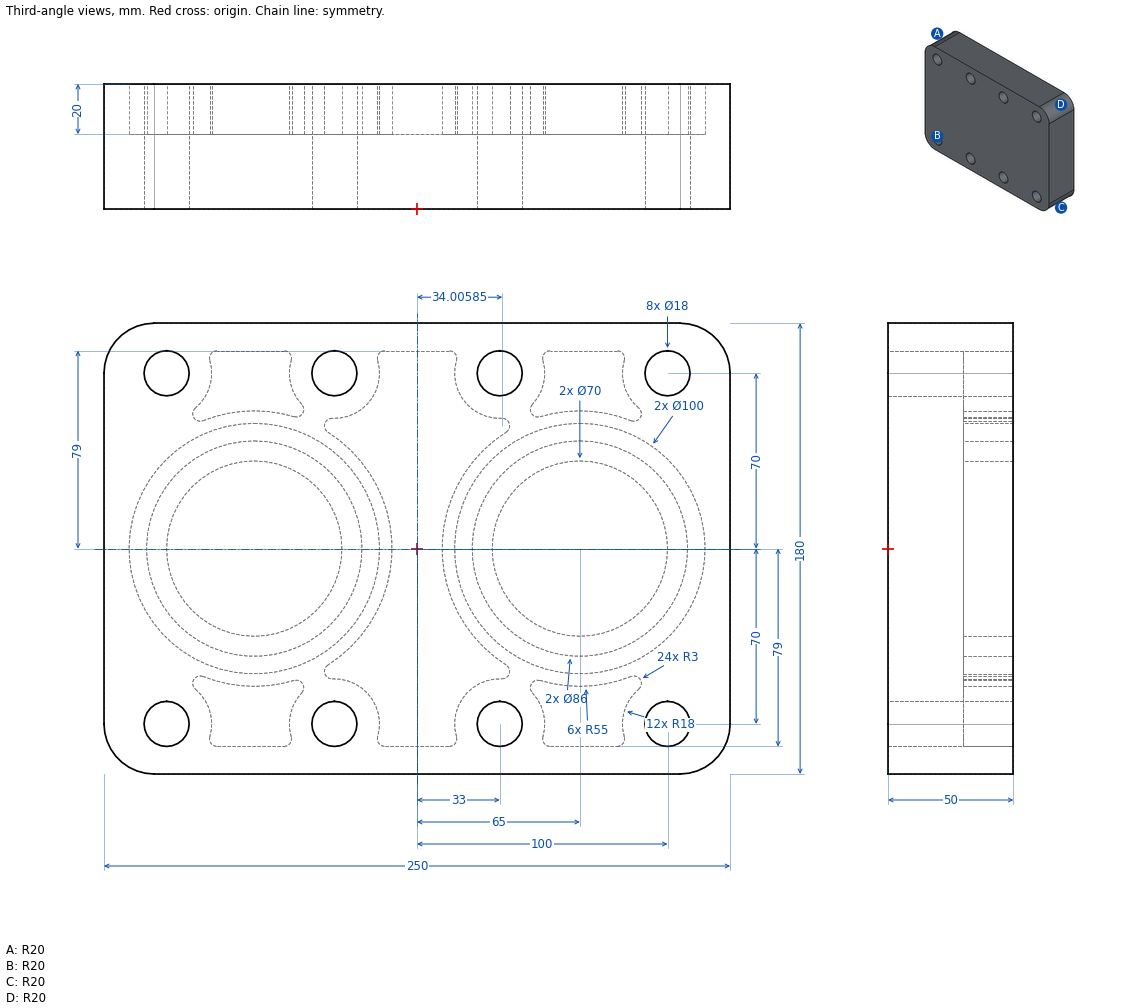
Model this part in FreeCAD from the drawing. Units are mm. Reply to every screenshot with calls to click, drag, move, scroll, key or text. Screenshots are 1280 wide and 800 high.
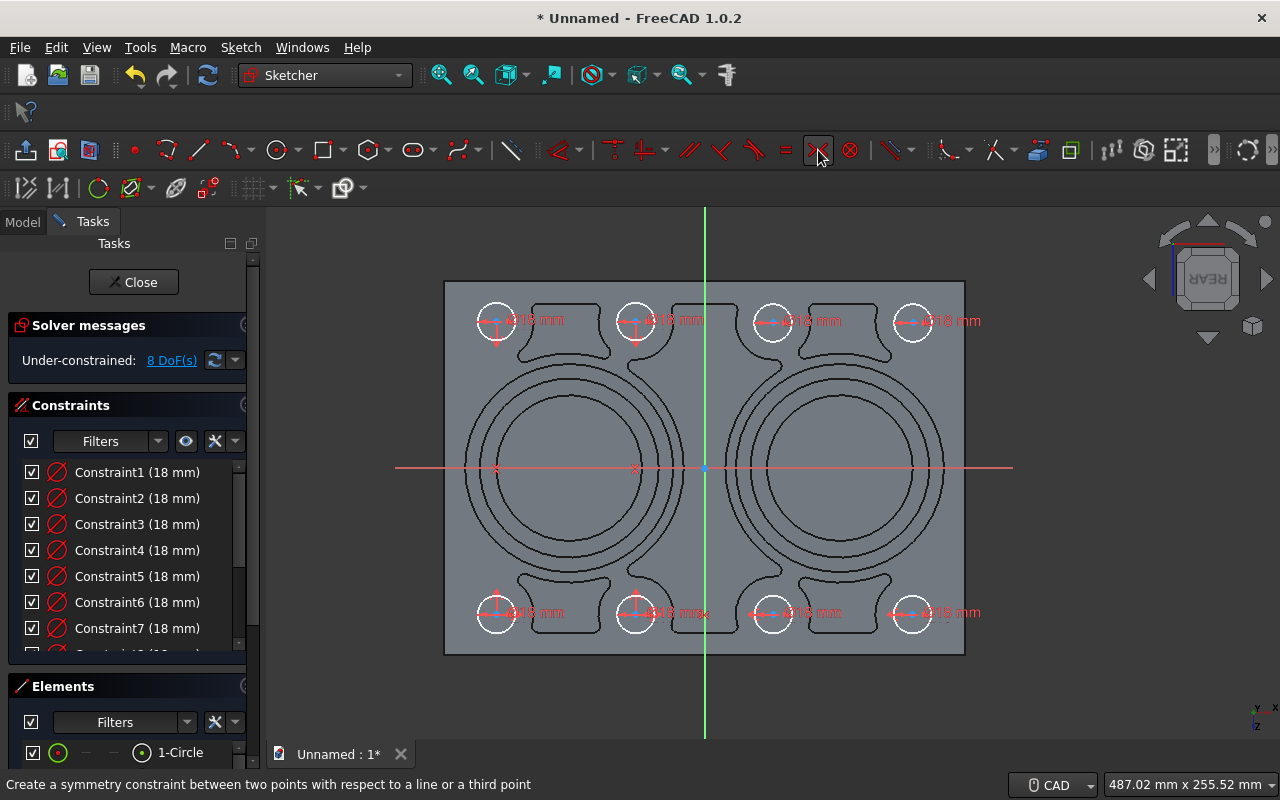
click(773, 615)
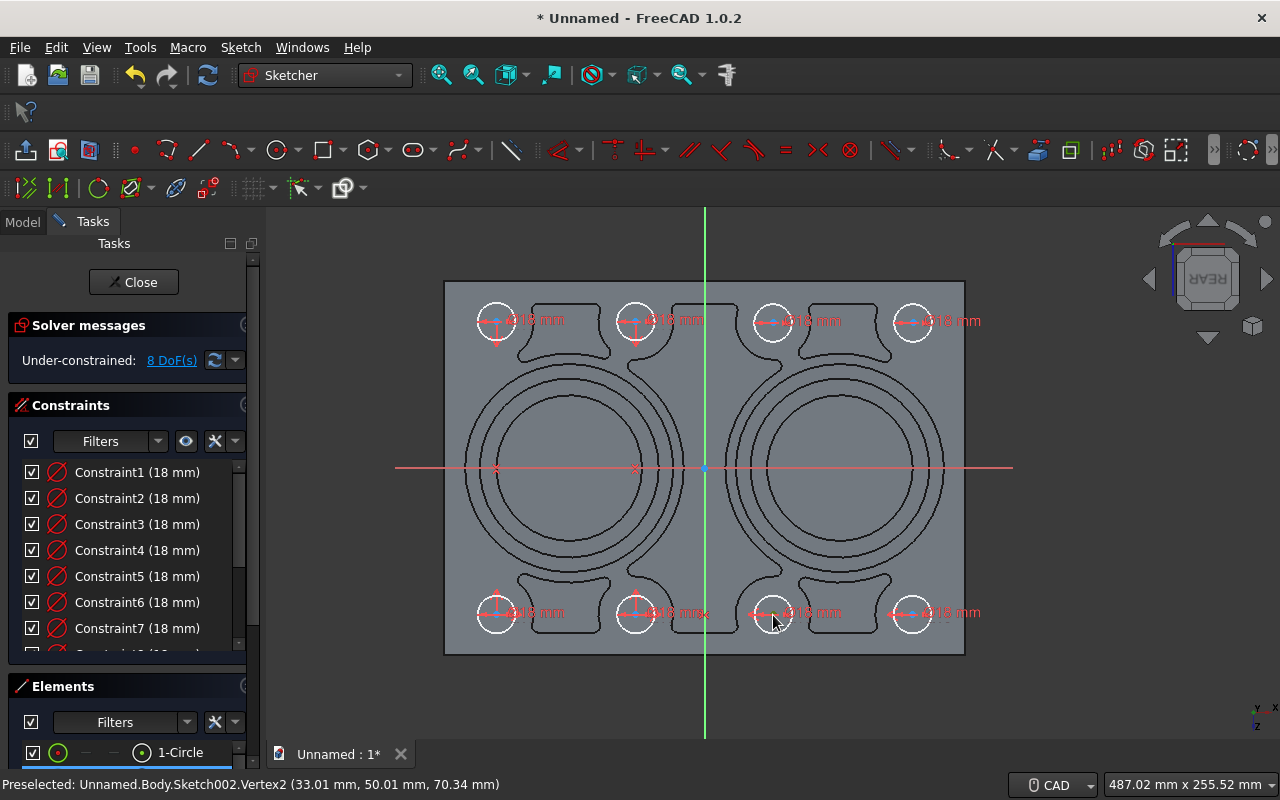
click(773, 323)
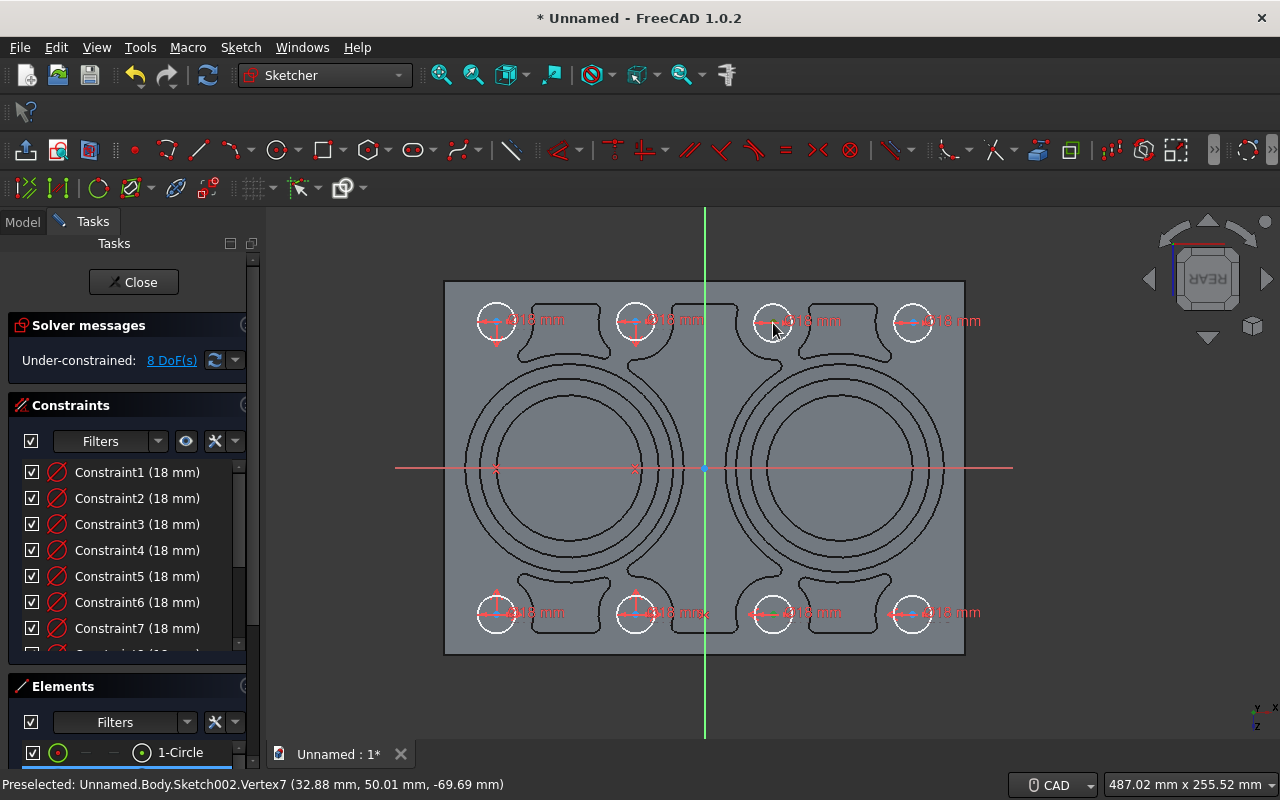
click(411, 468)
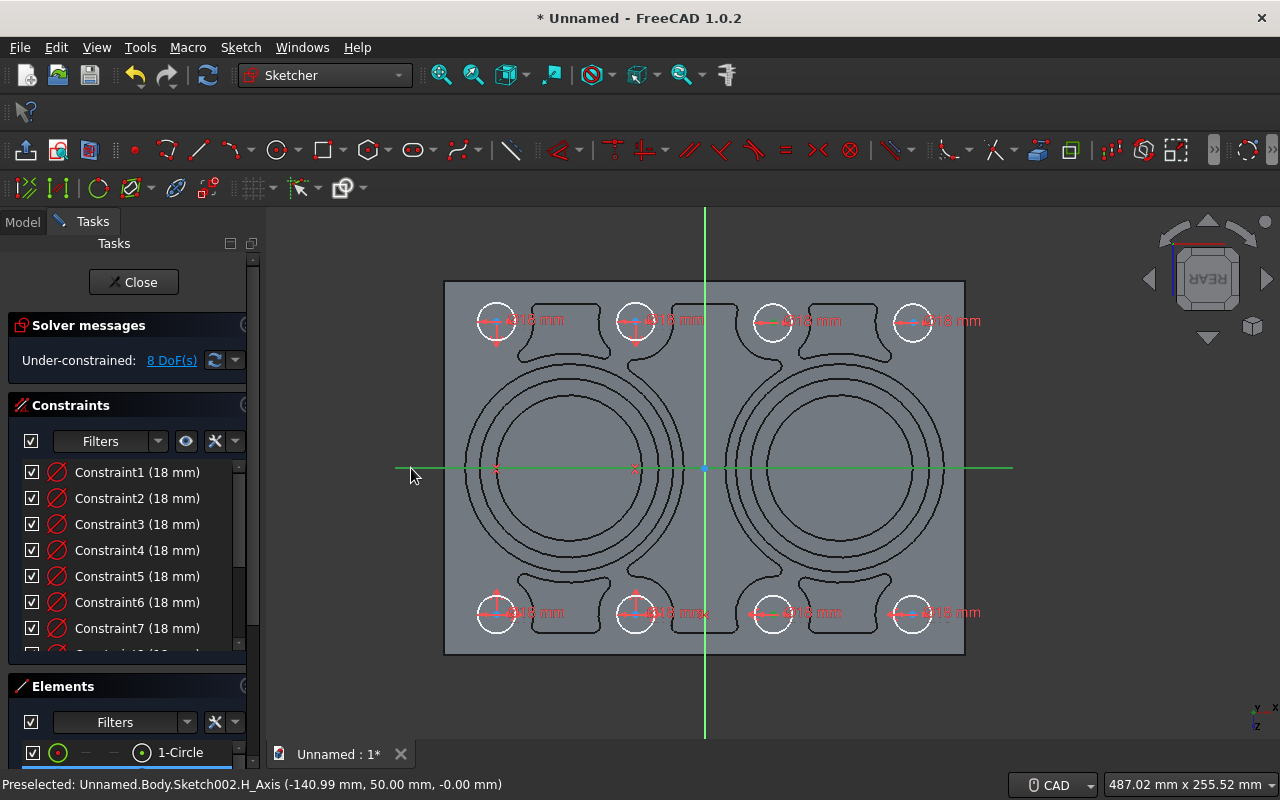
click(818, 150)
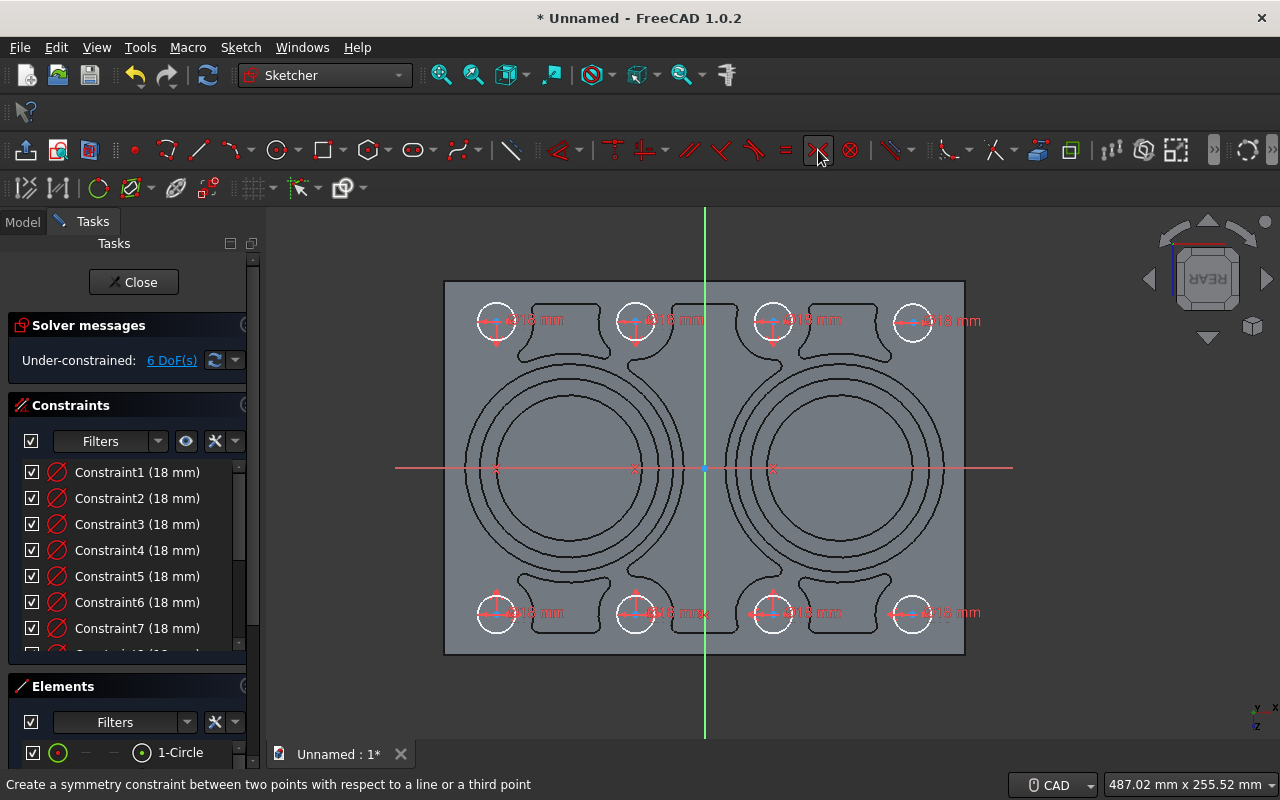
click(913, 615)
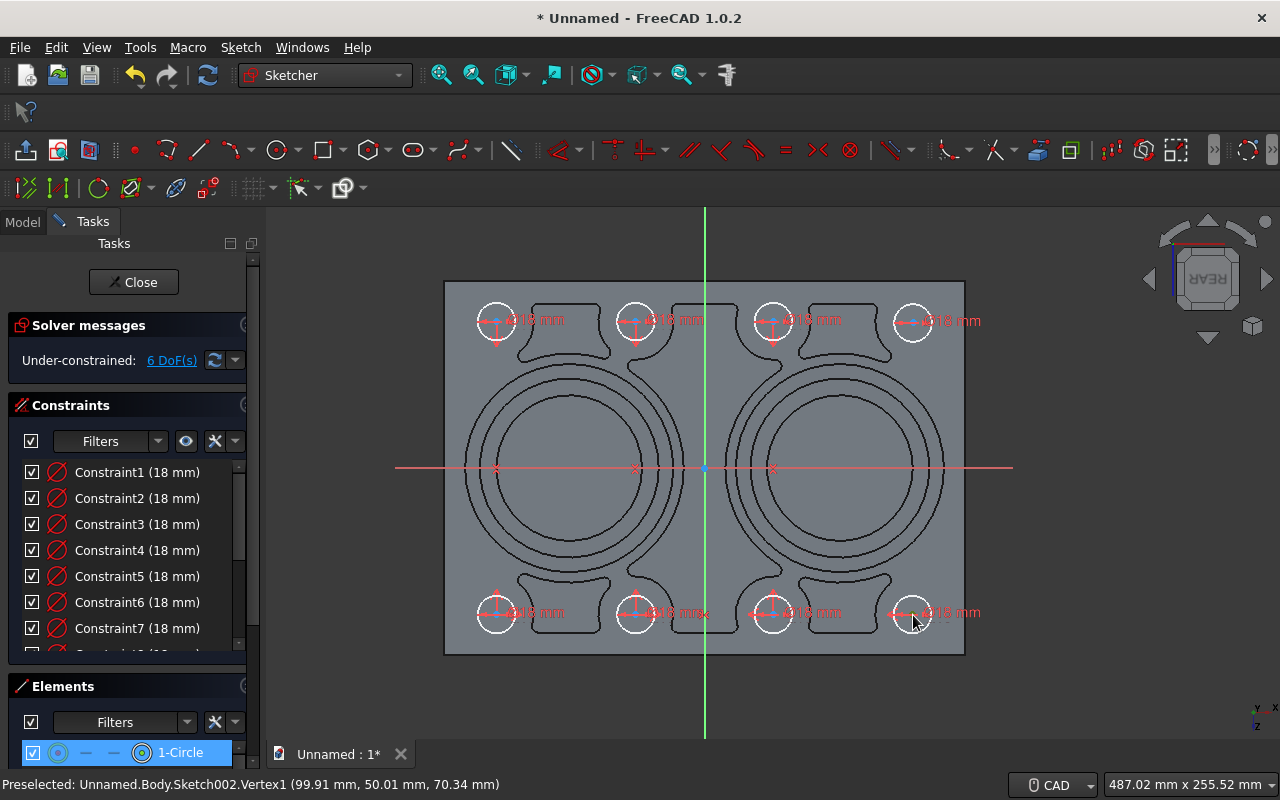
click(913, 323)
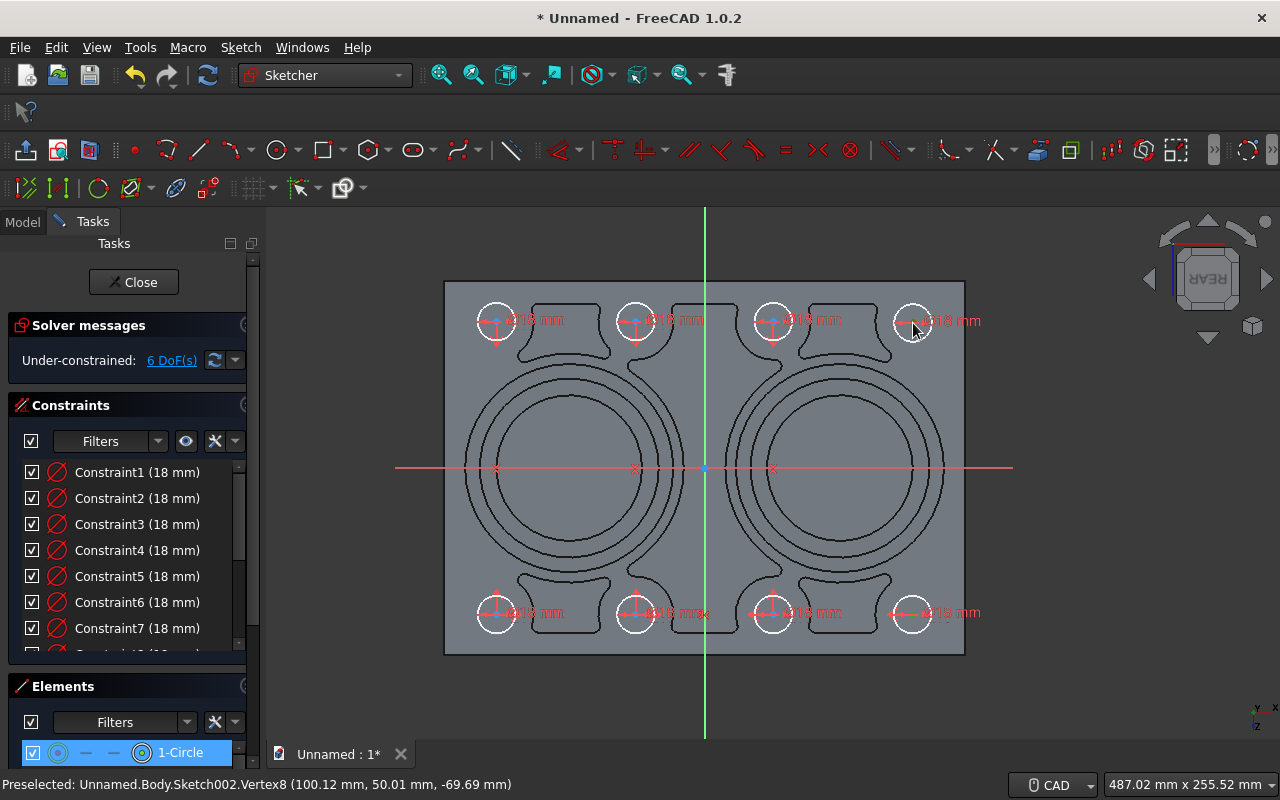
click(411, 468)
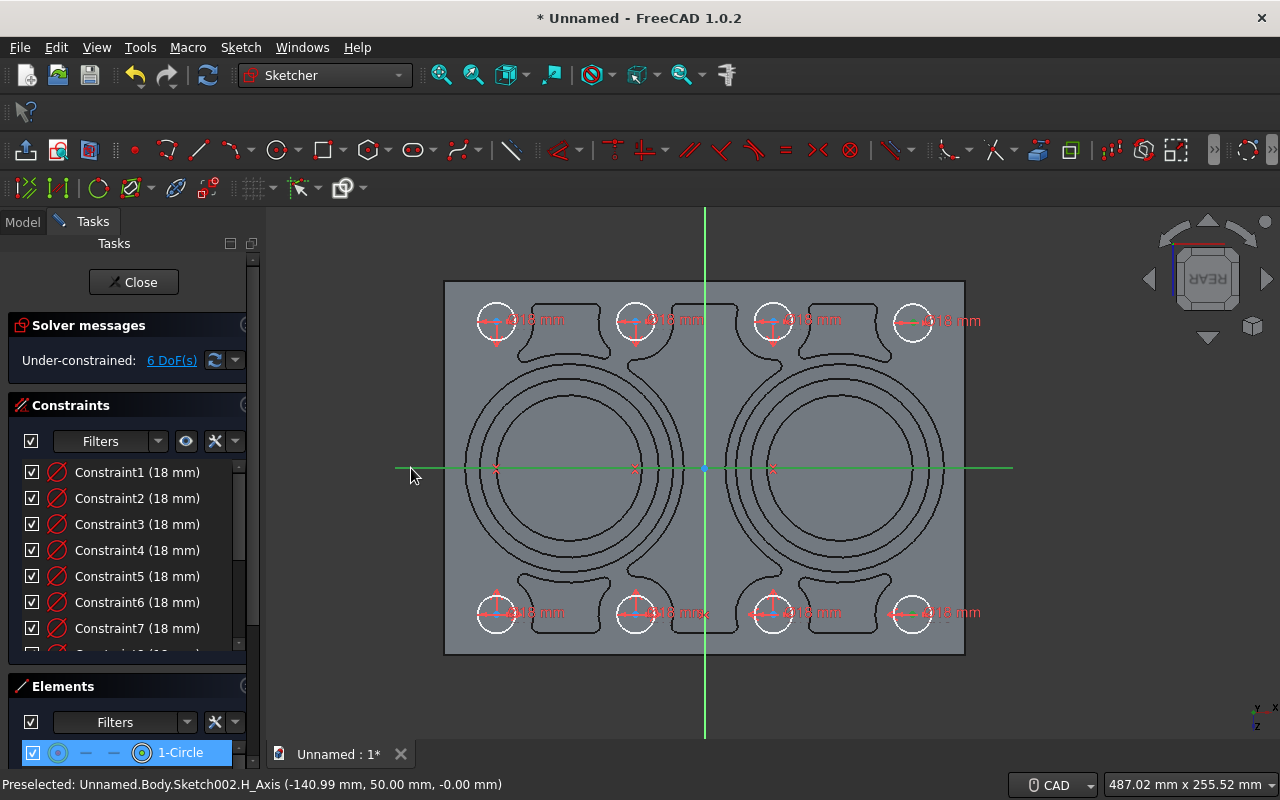
click(818, 150)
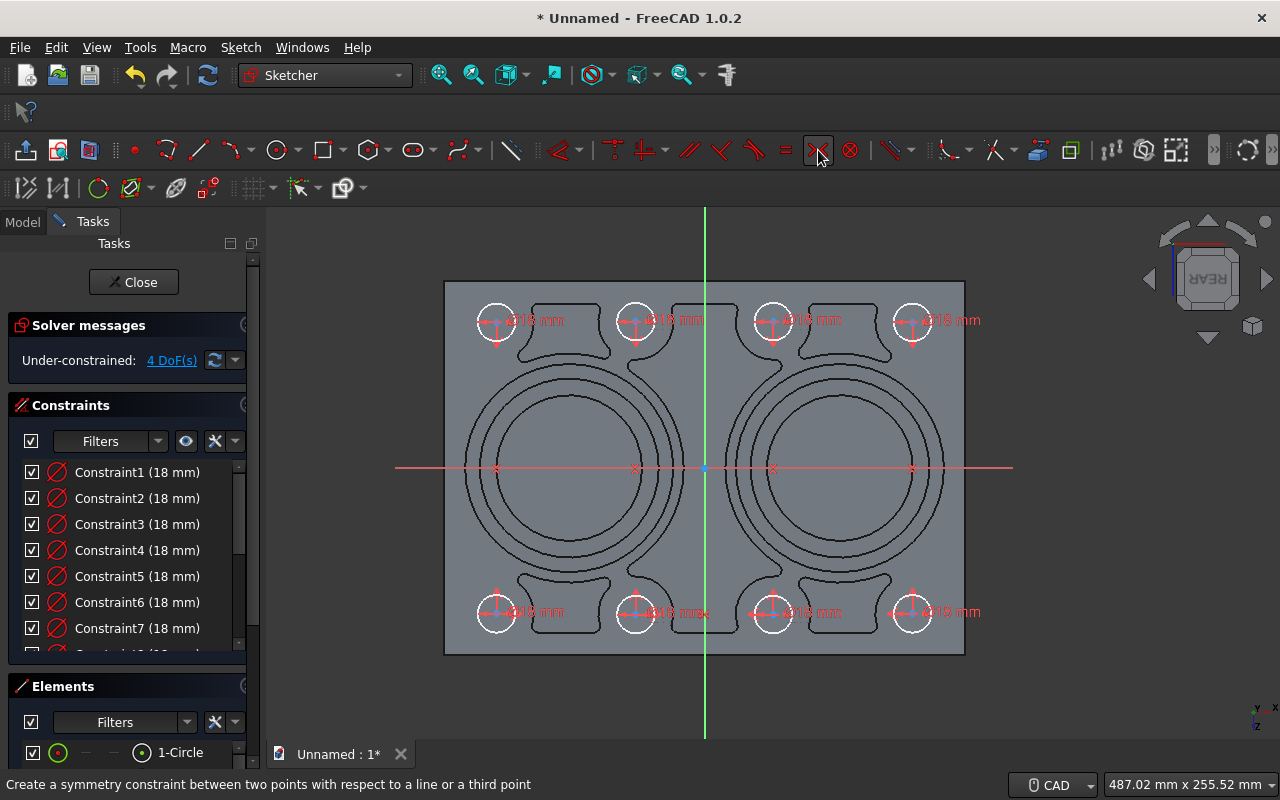
click(558, 150)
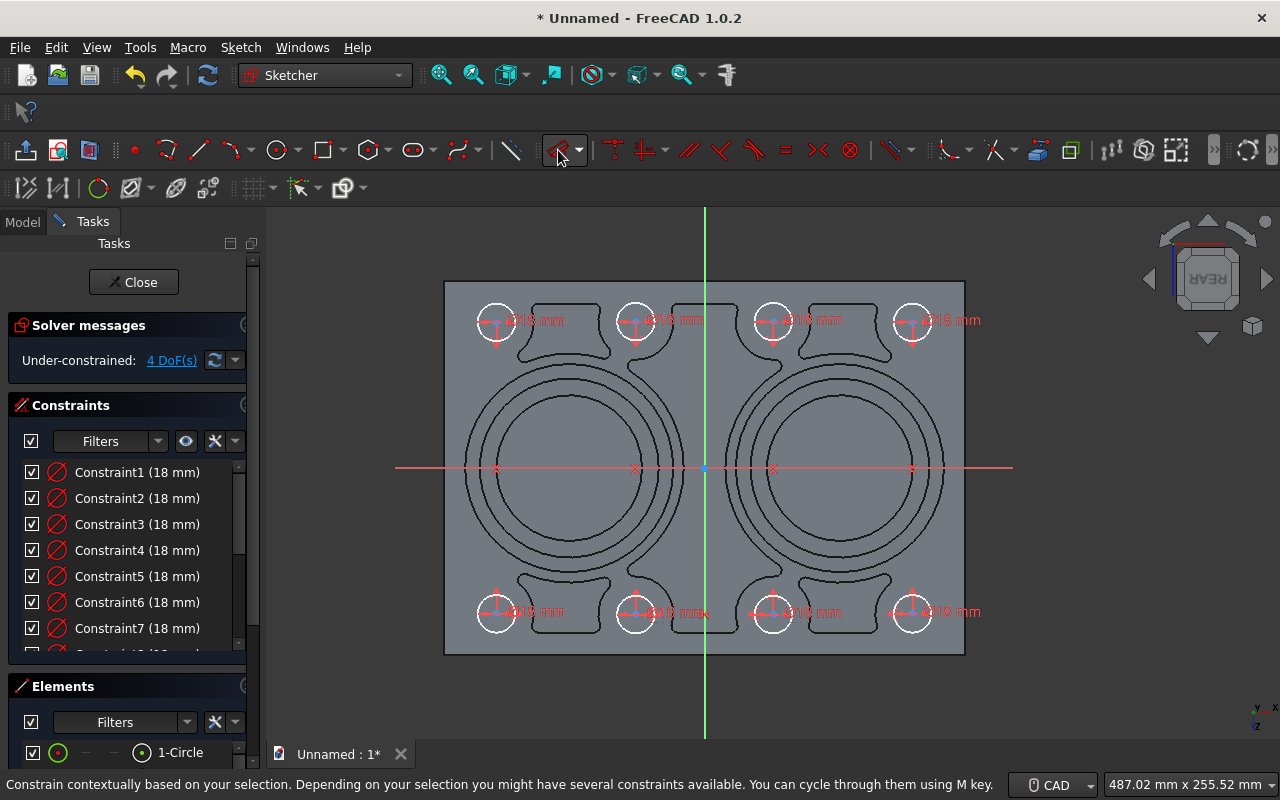
click(913, 614)
click(947, 541)